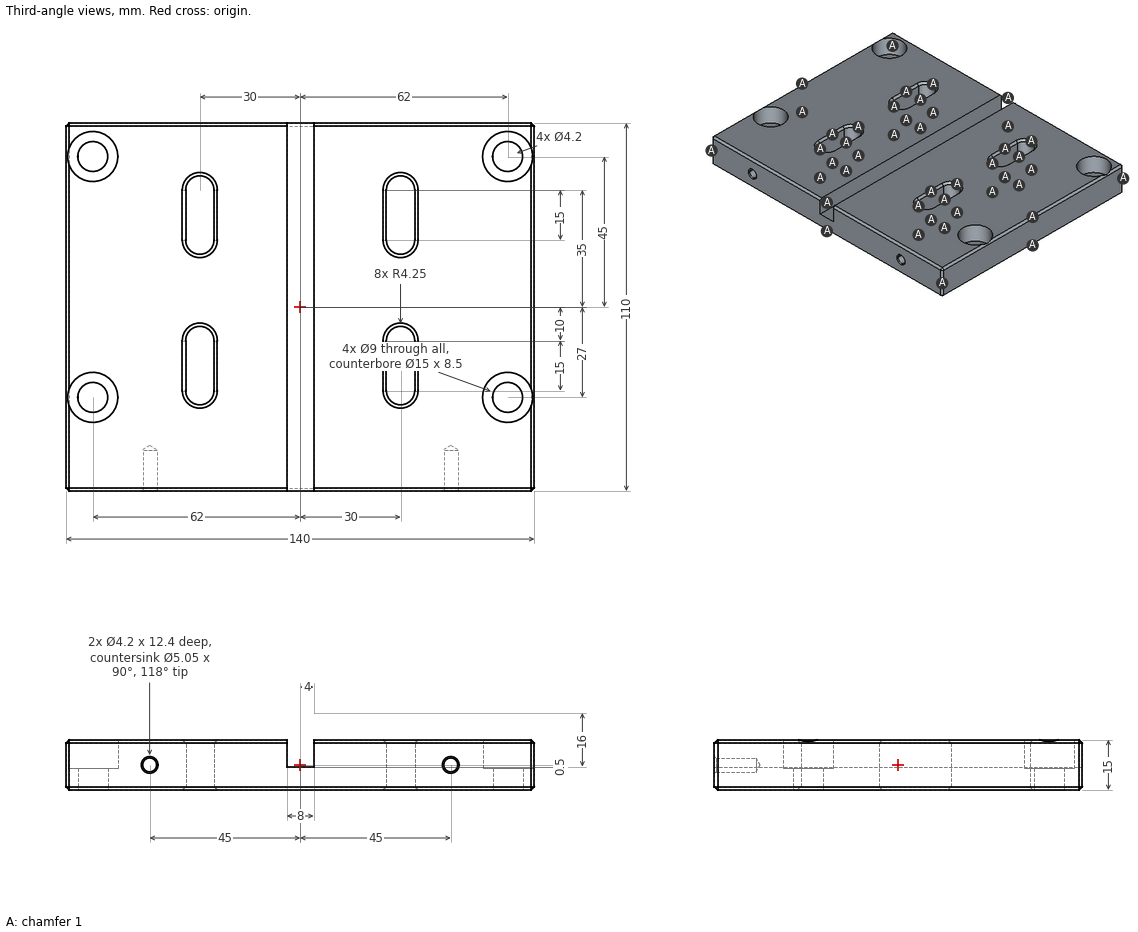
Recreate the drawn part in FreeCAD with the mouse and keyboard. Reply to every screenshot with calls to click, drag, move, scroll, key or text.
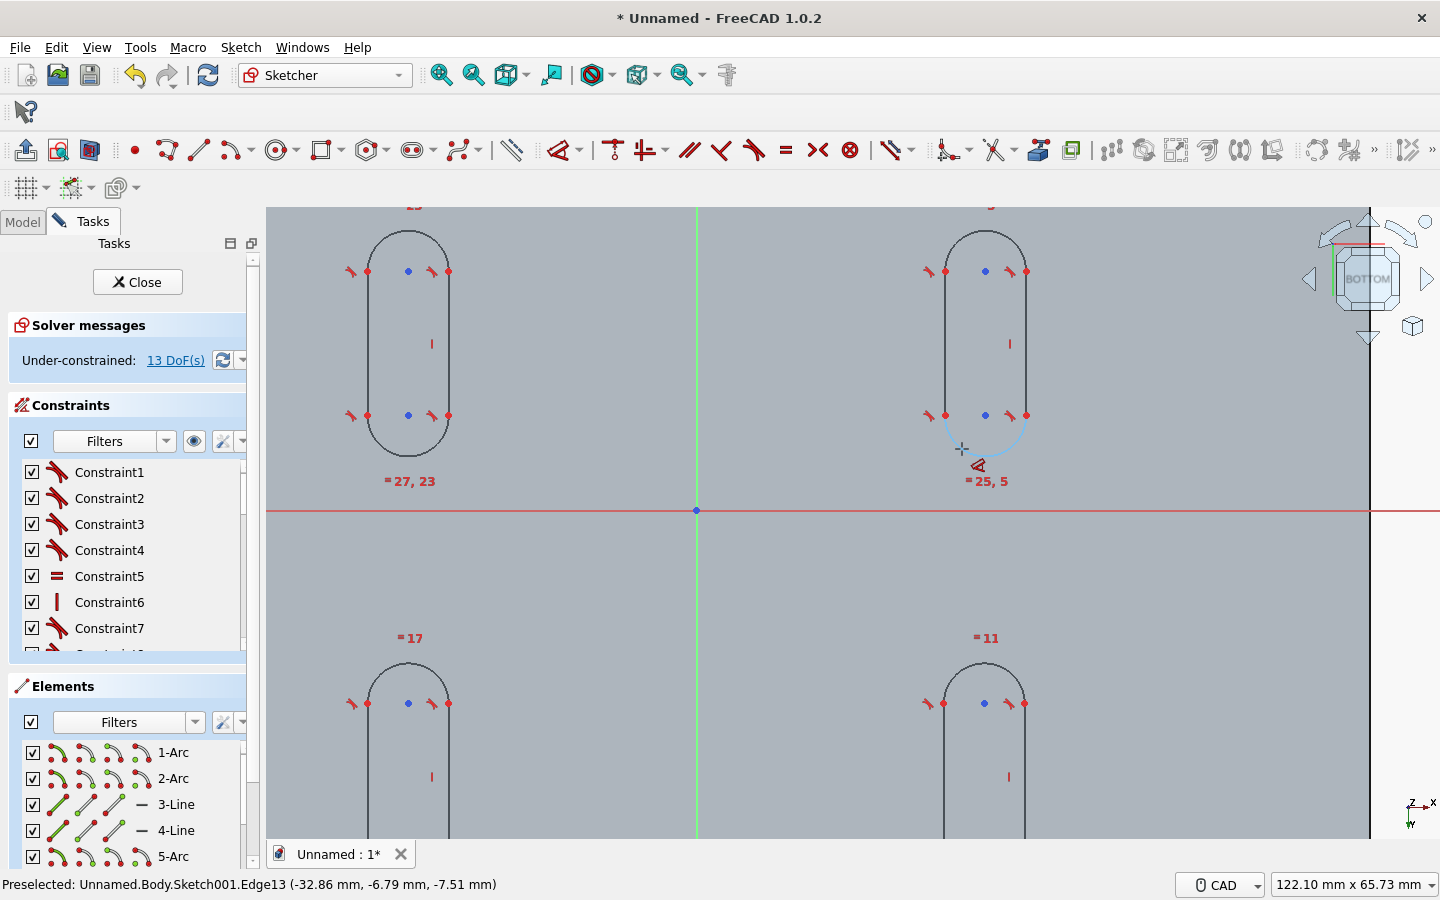
click(962, 449)
click(943, 475)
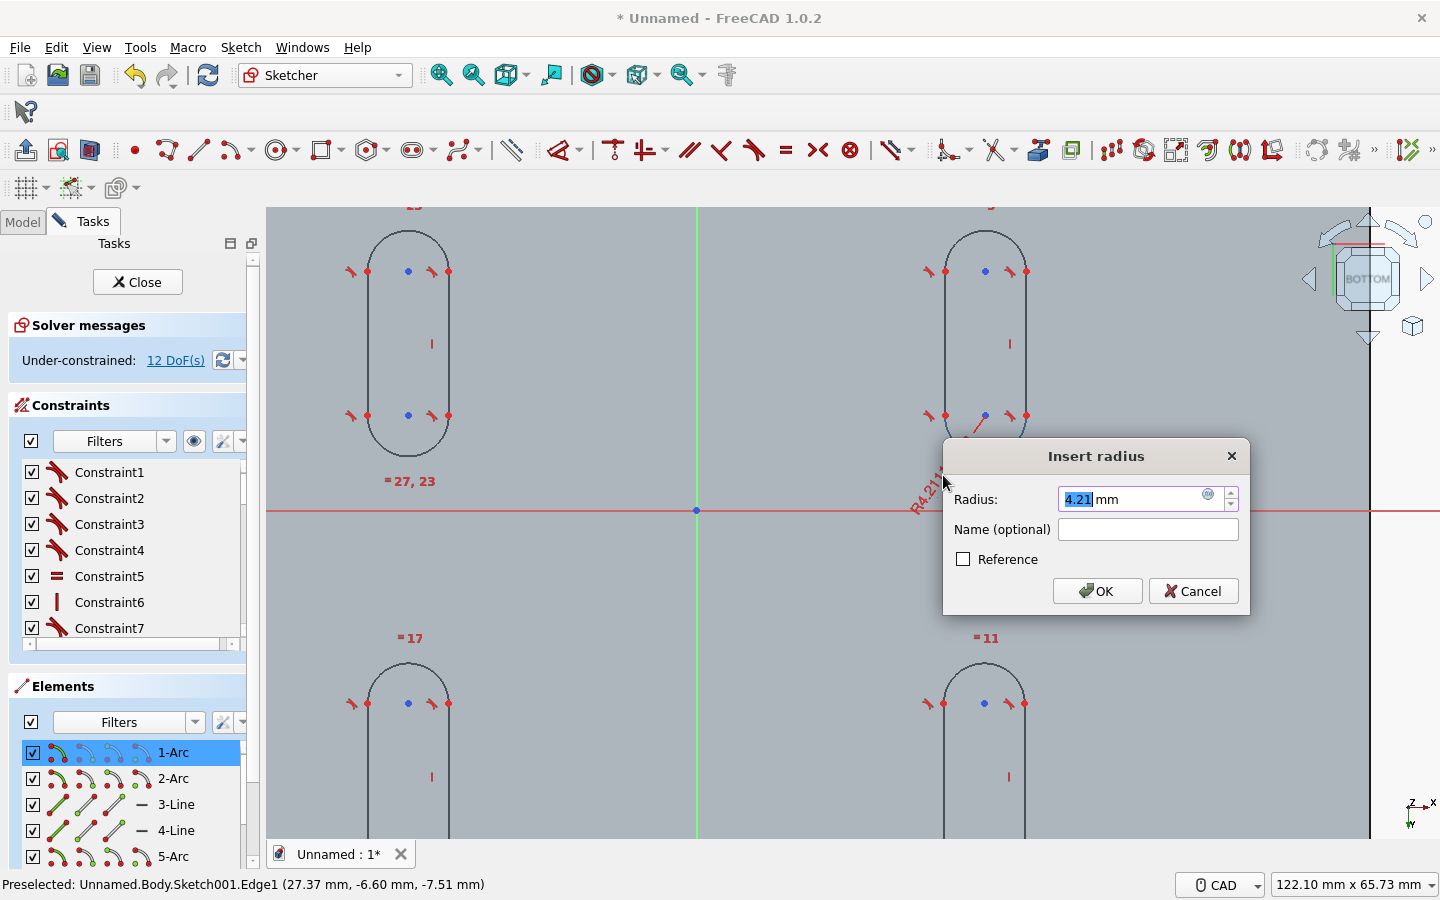
text(4.25)
key(Return)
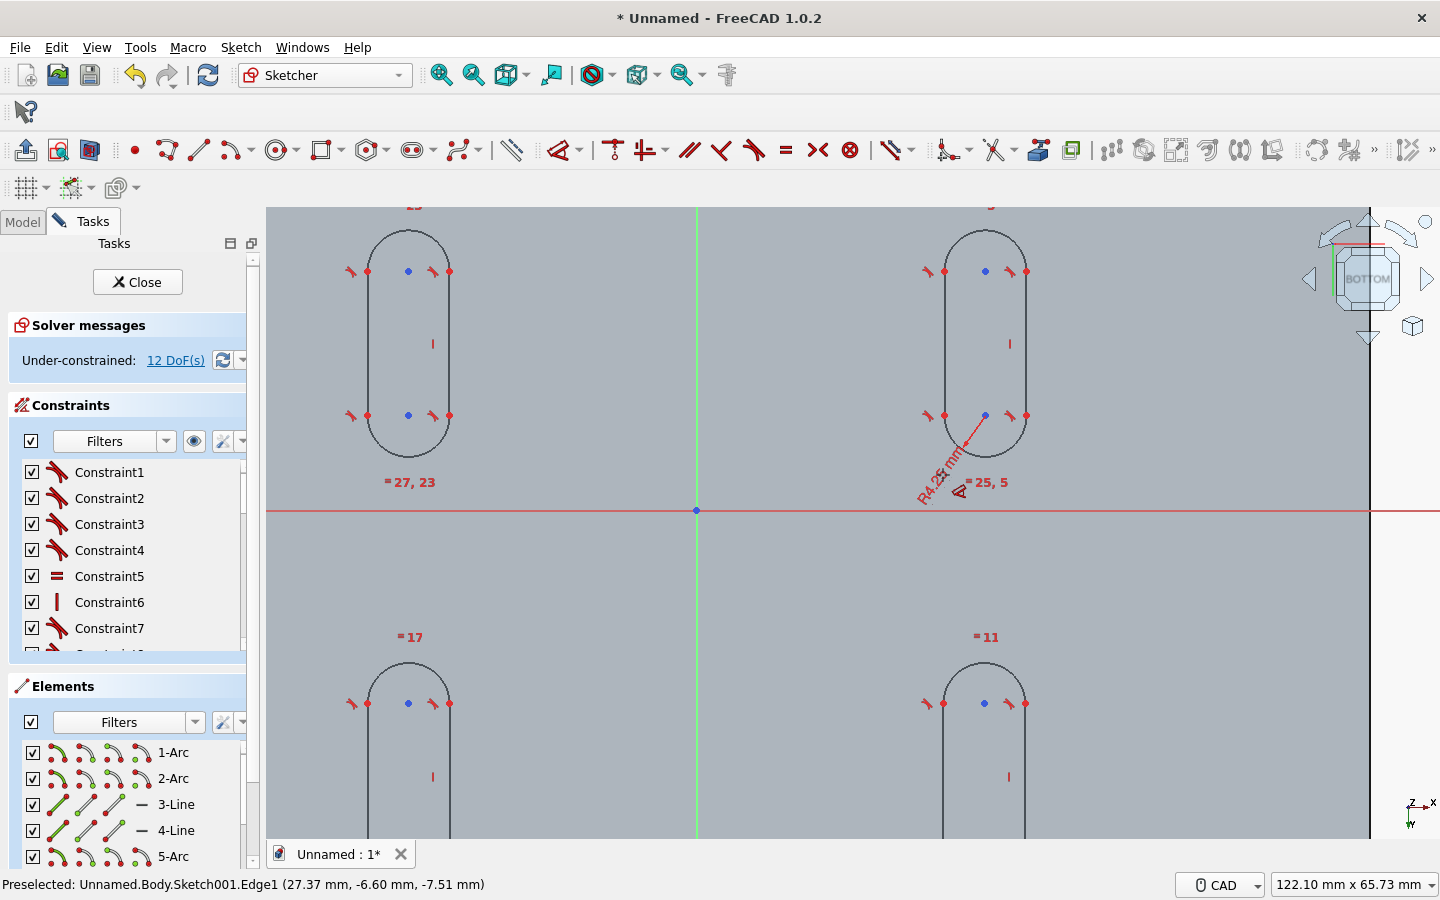
click(945, 373)
click(979, 344)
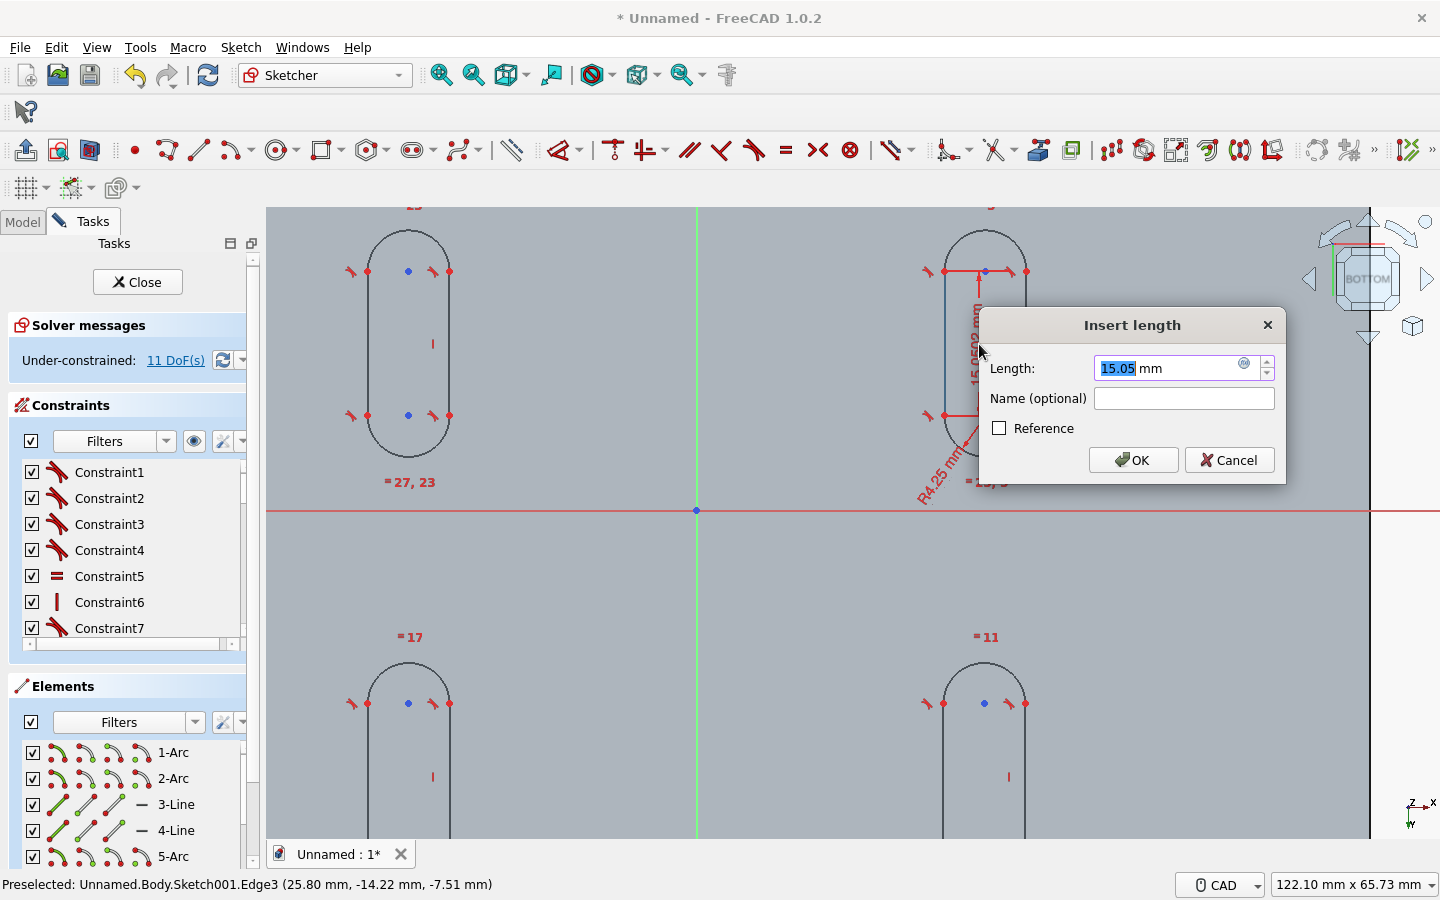
text(15)
key(Return)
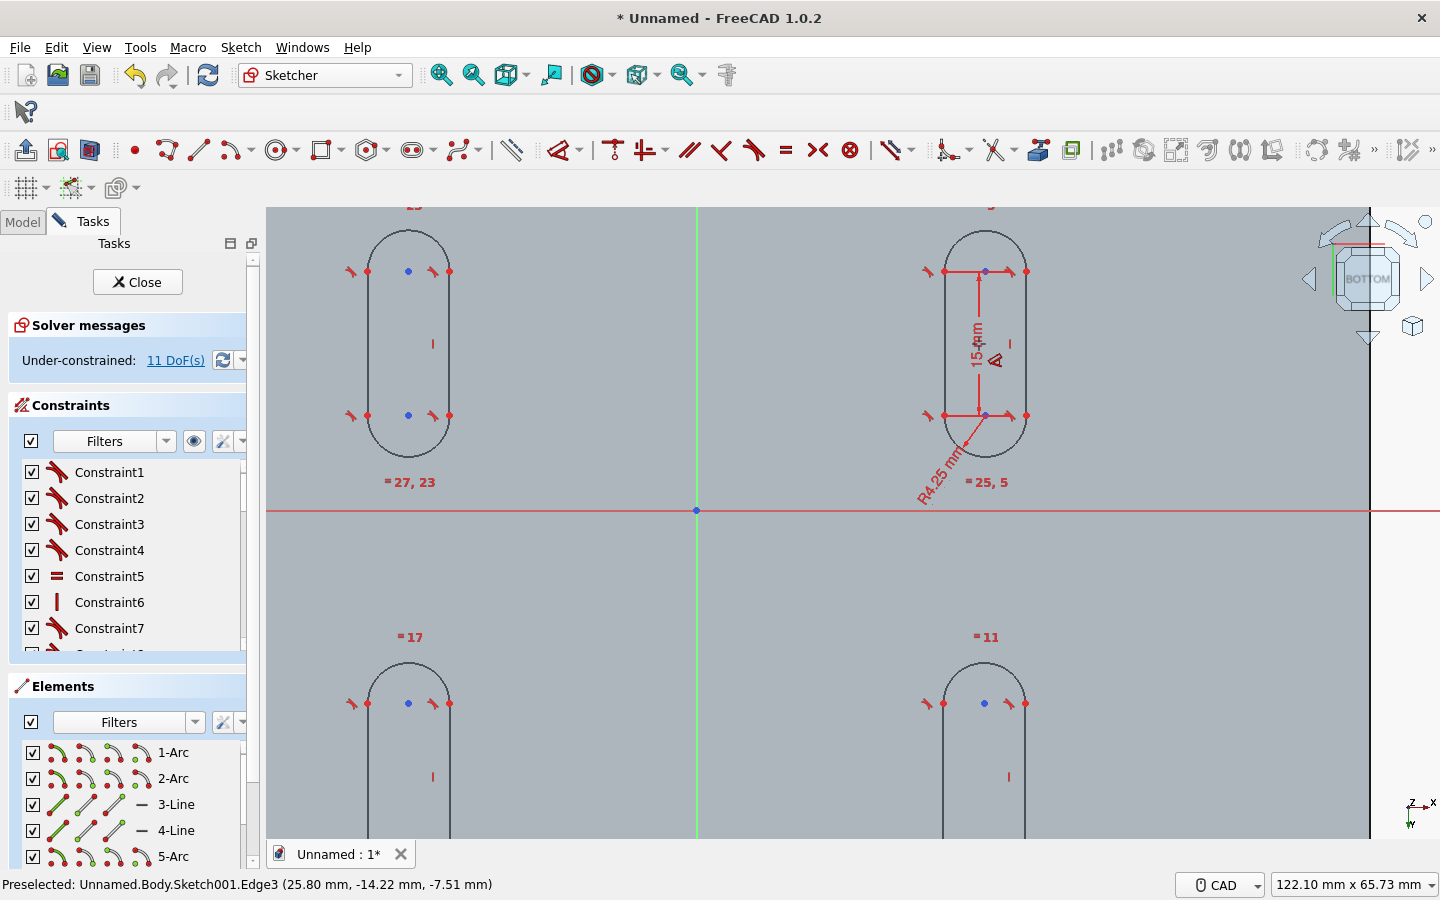
click(943, 805)
click(977, 757)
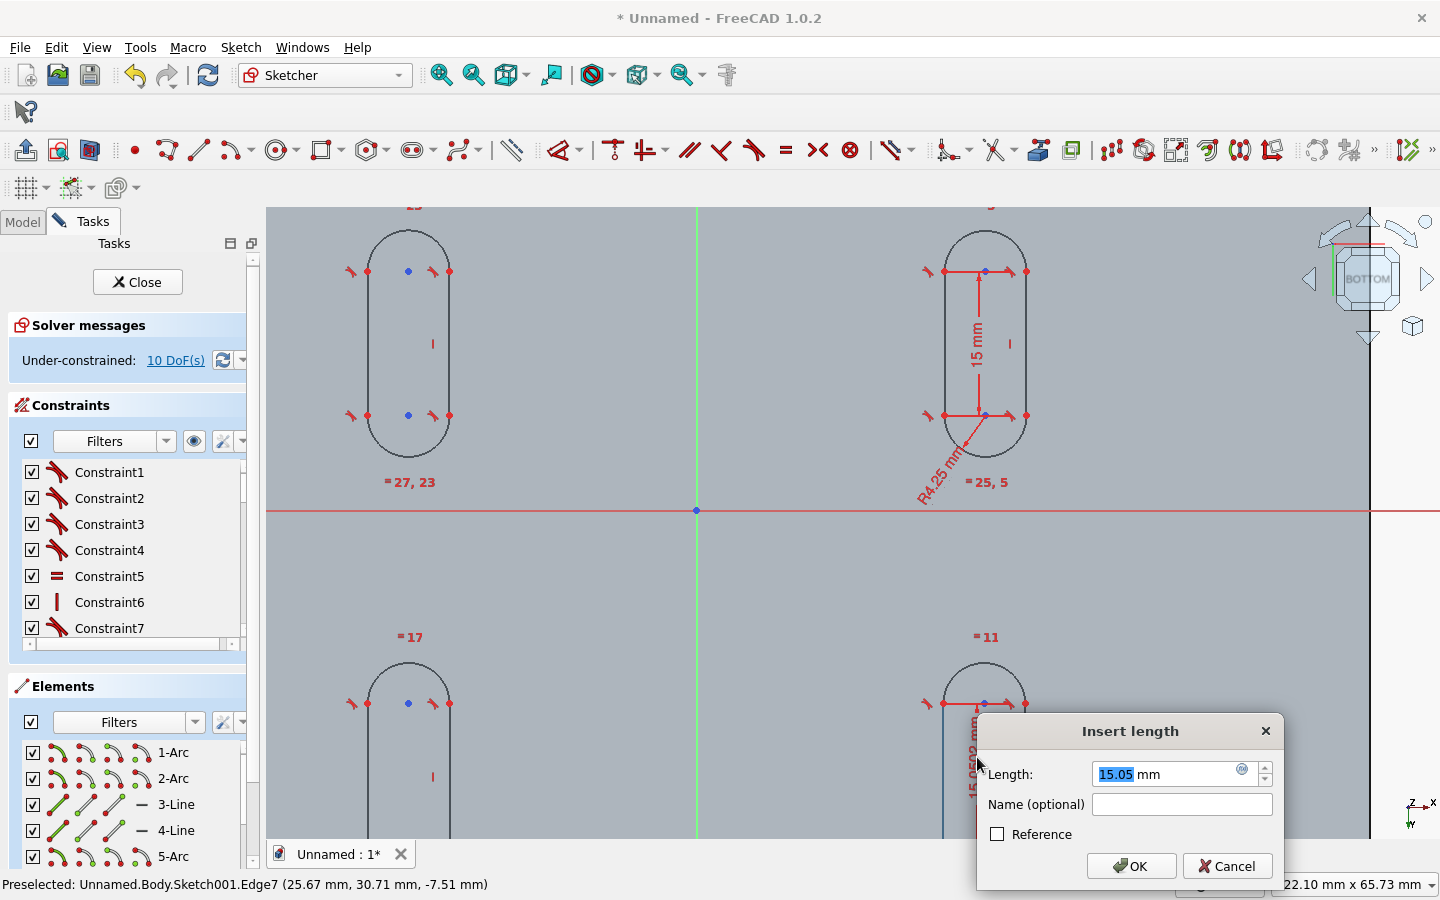
text(15)
key(Return)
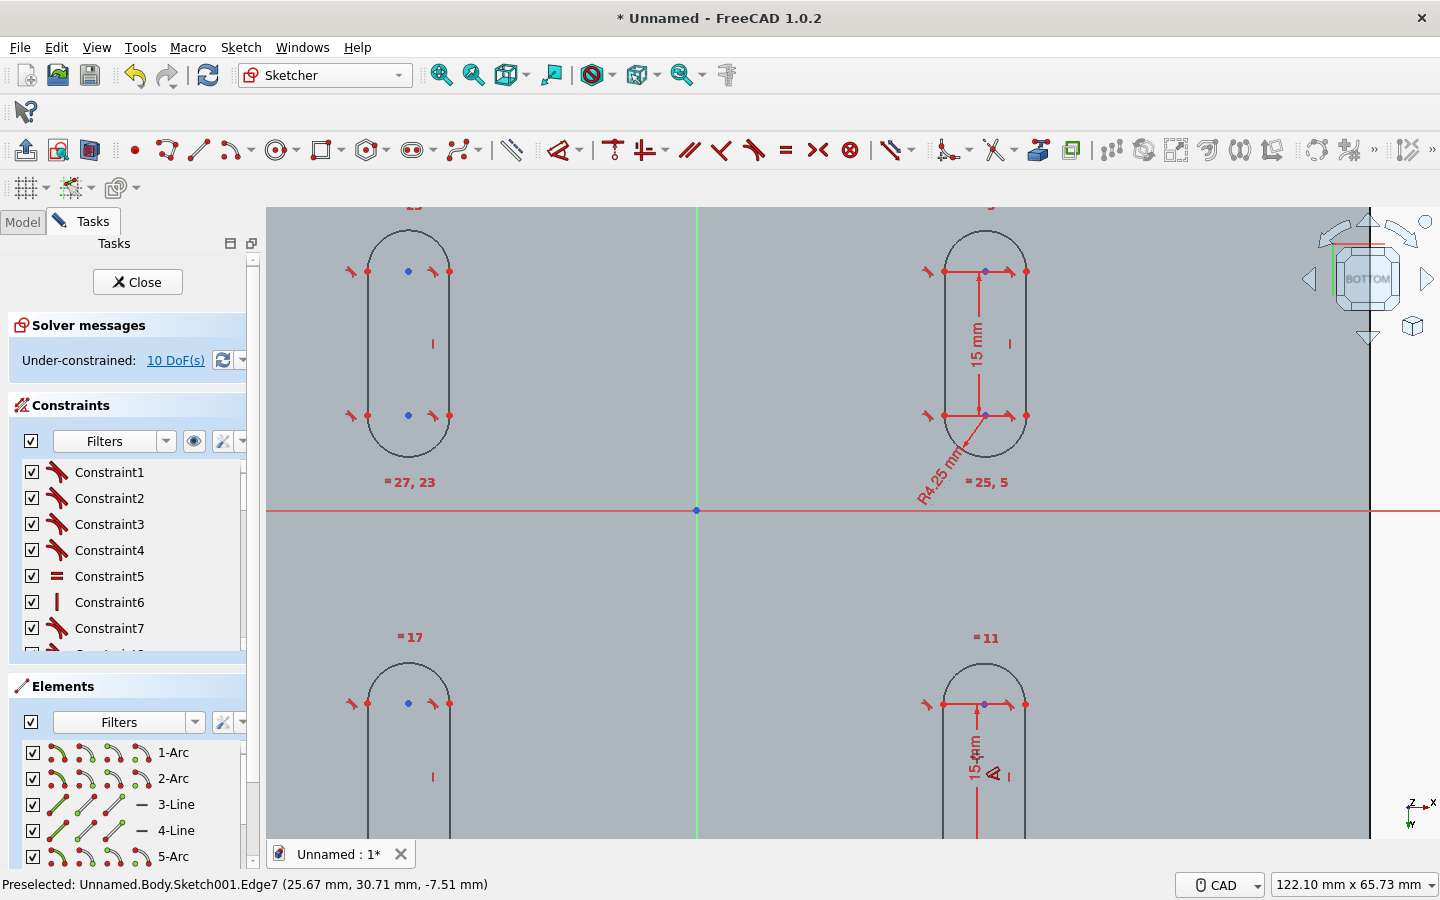
click(368, 805)
click(334, 757)